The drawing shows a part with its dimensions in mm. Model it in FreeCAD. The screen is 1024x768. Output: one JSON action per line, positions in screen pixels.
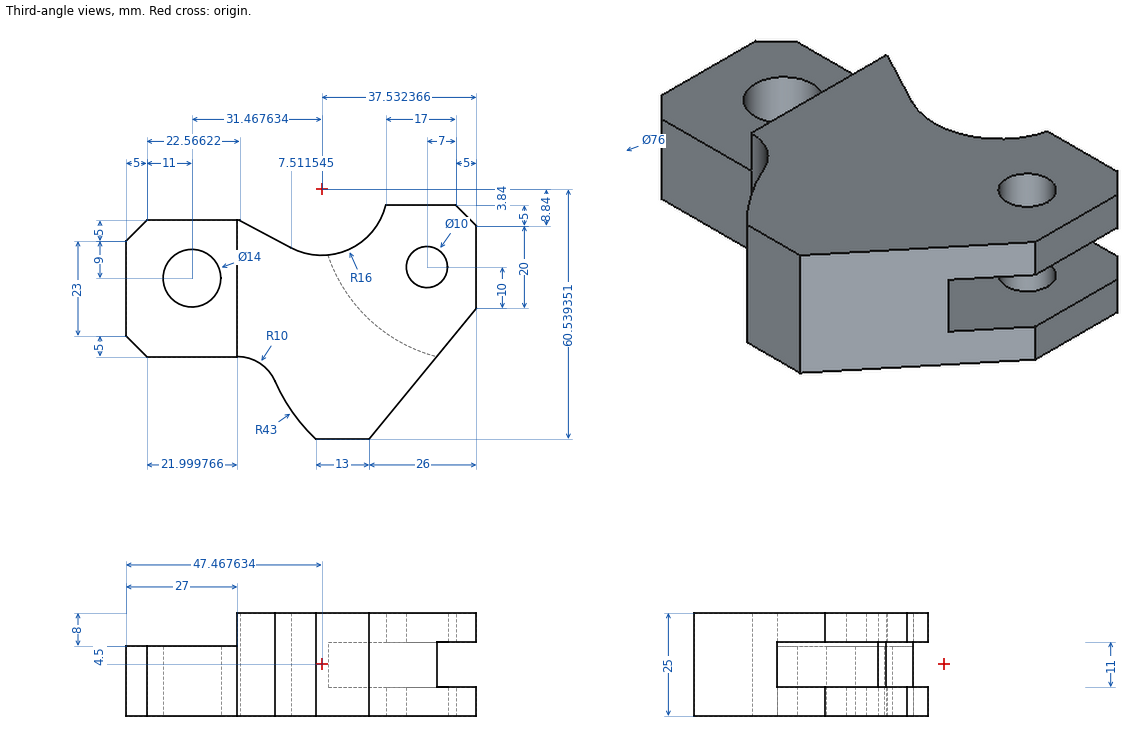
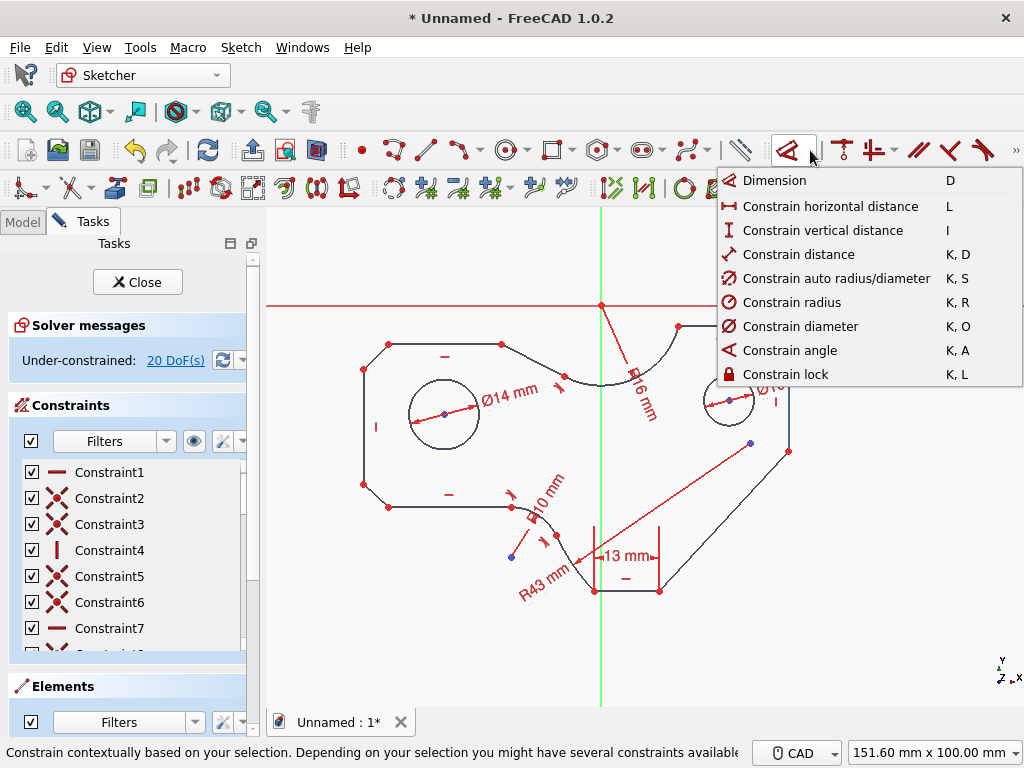
{"action": "left_click", "coordinate": [870, 230]}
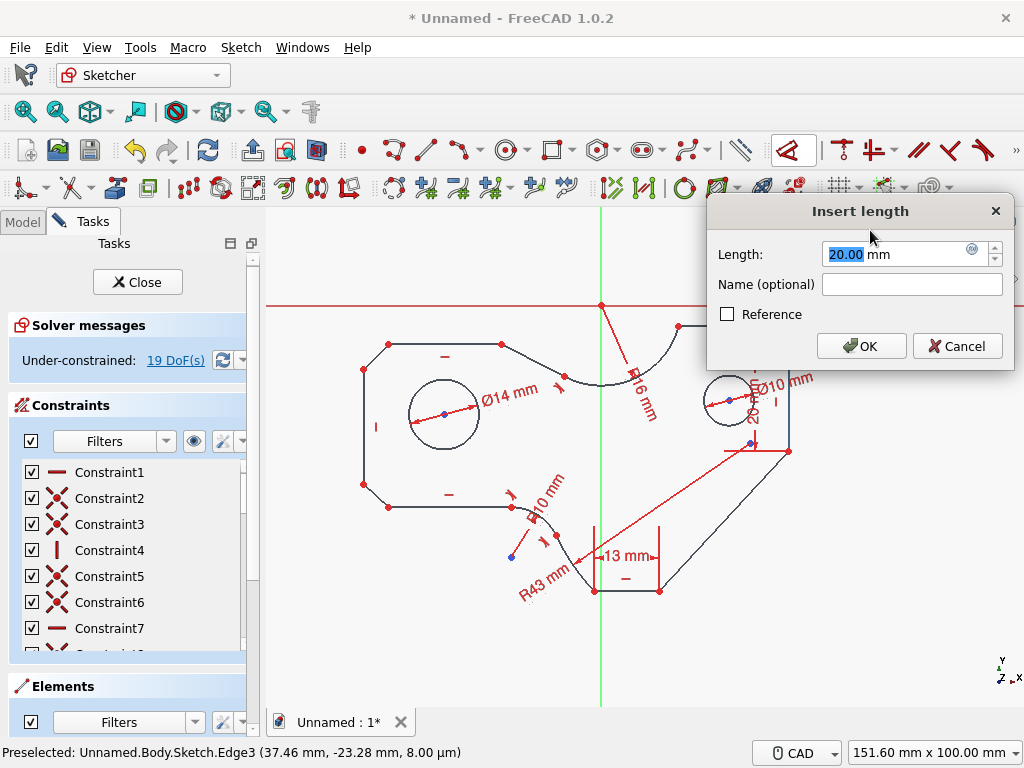
{"action": "type", "text": "20"}
{"action": "key", "text": "Return"}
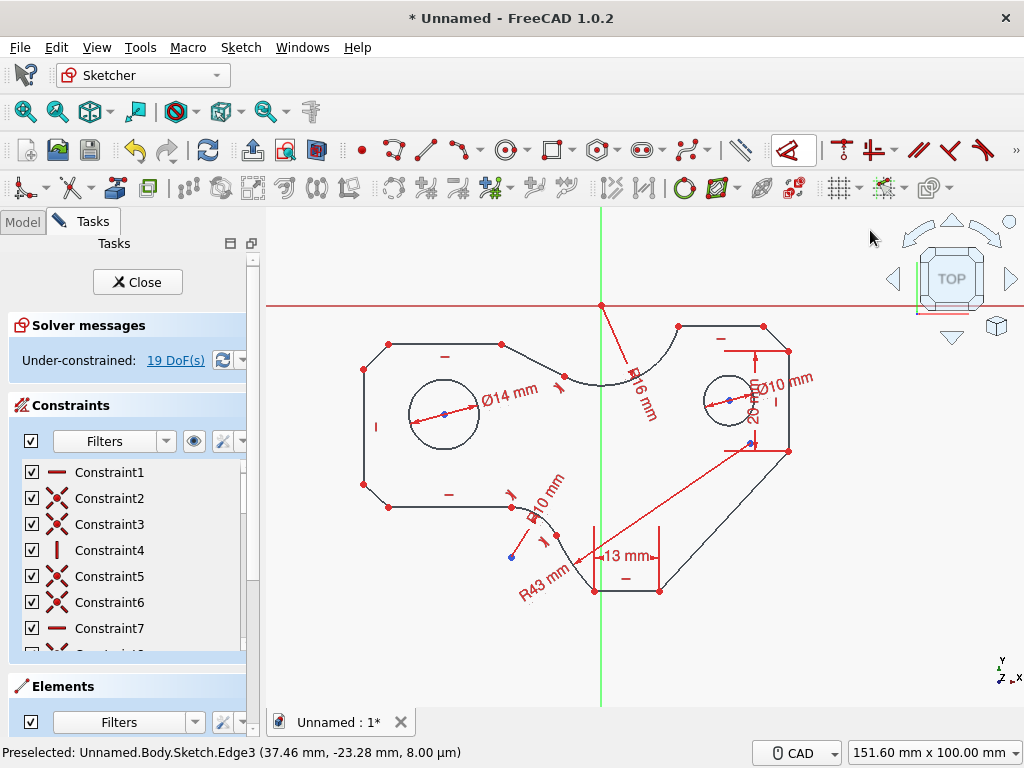
{"action": "left_click", "coordinate": [738, 326]}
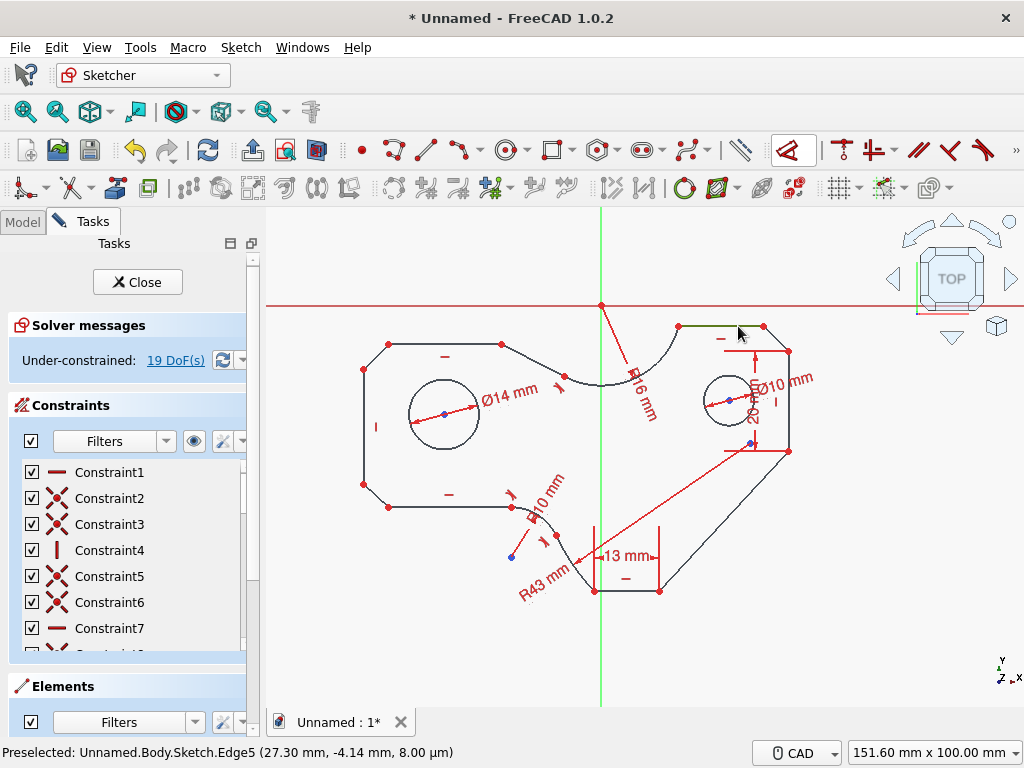
{"action": "left_click", "coordinate": [810, 150]}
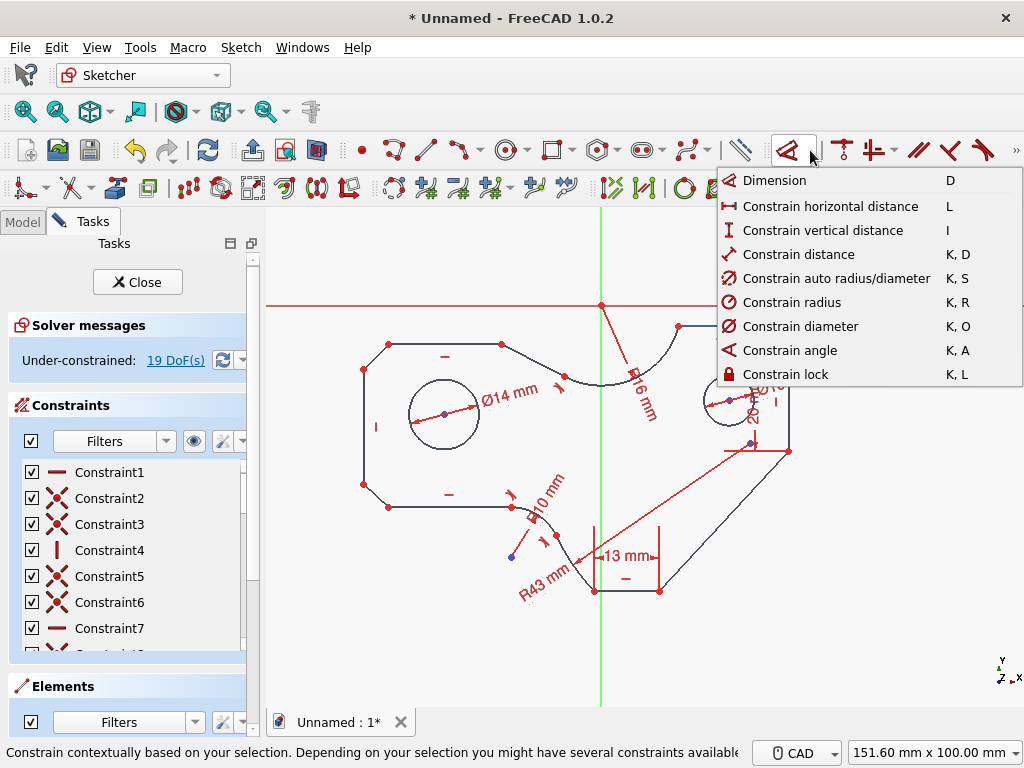
{"action": "left_click", "coordinate": [870, 206]}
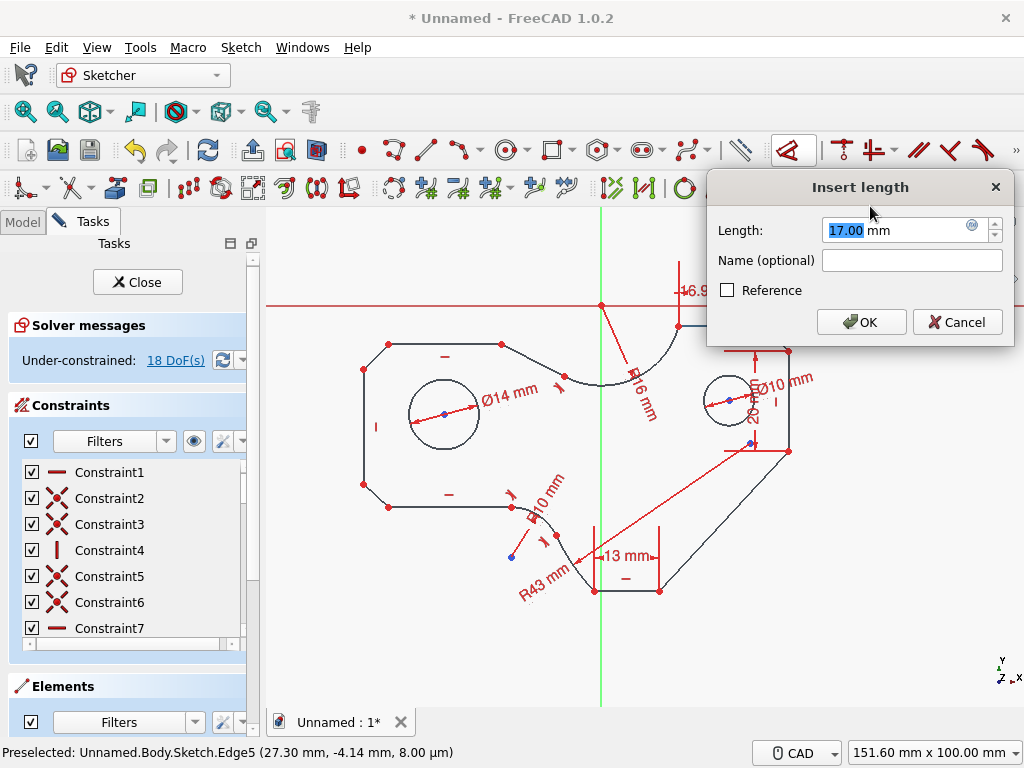
{"action": "type", "text": "17"}
{"action": "key", "text": "Return"}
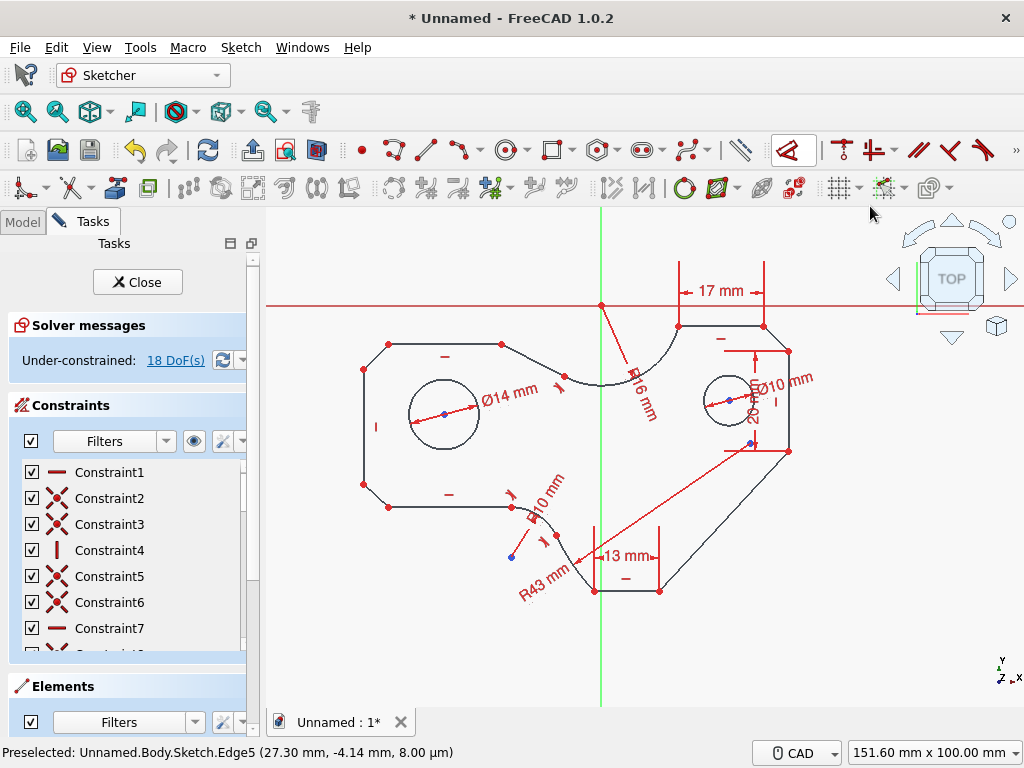
{"action": "left_click", "coordinate": [364, 404]}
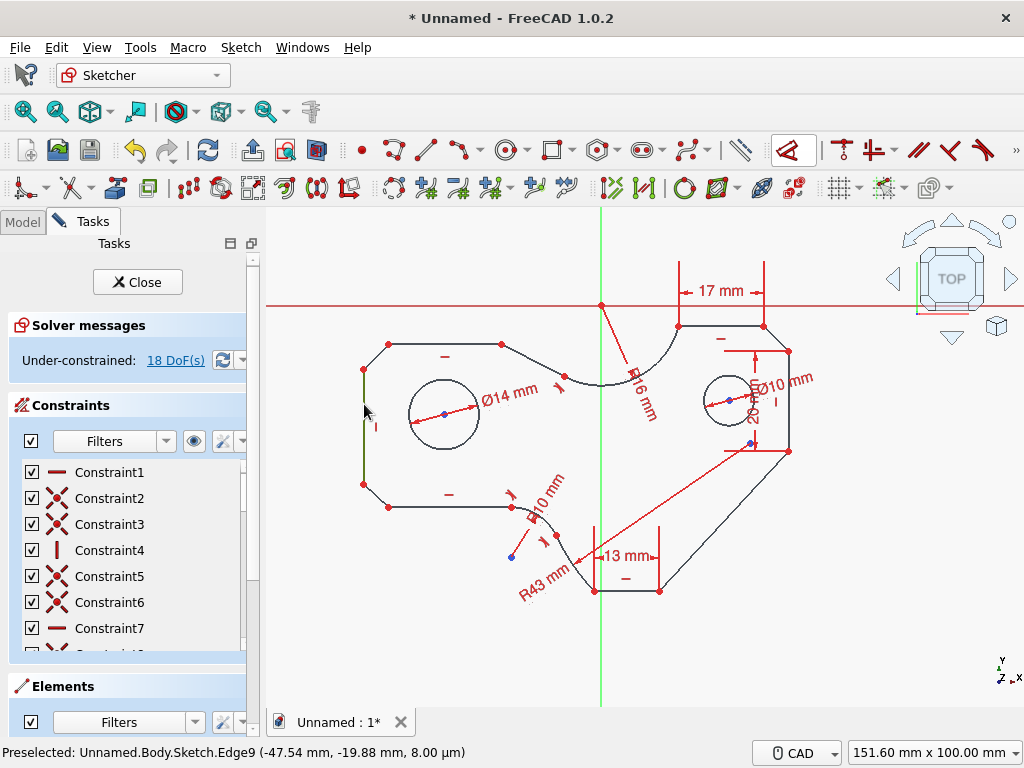
{"action": "key", "text": "i"}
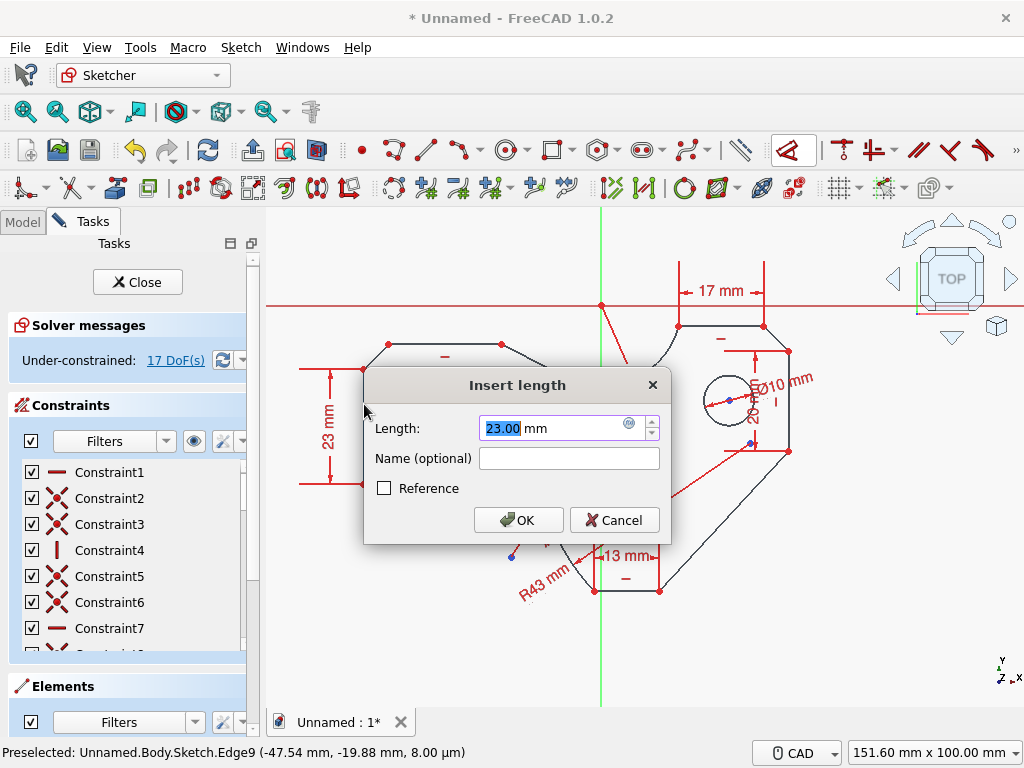
{"action": "type", "text": "23"}
{"action": "key", "text": "Return"}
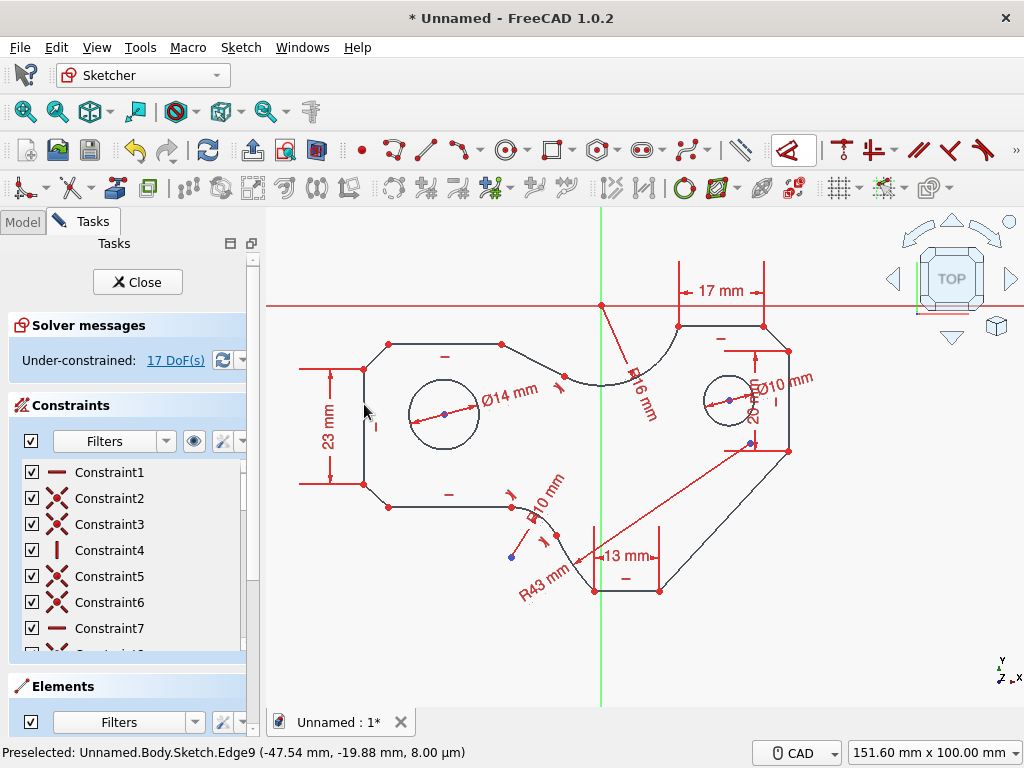
{"action": "scroll", "coordinate": [781, 344], "scroll_direction": "up", "scroll_amount": 3}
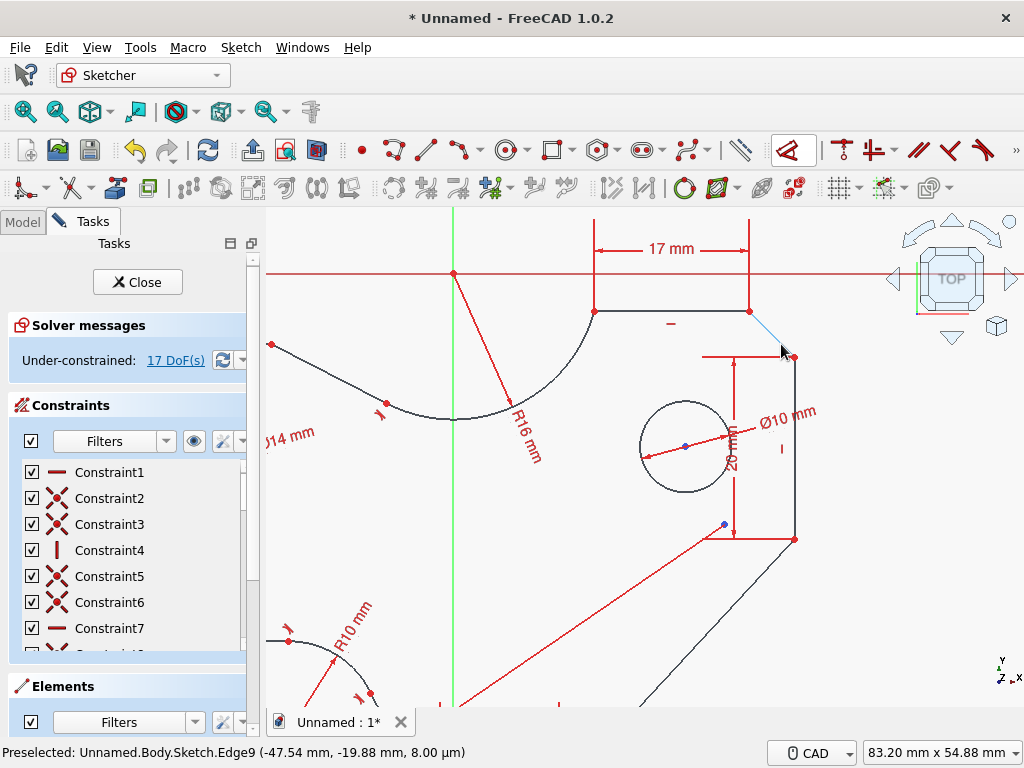
{"action": "left_click", "coordinate": [781, 343]}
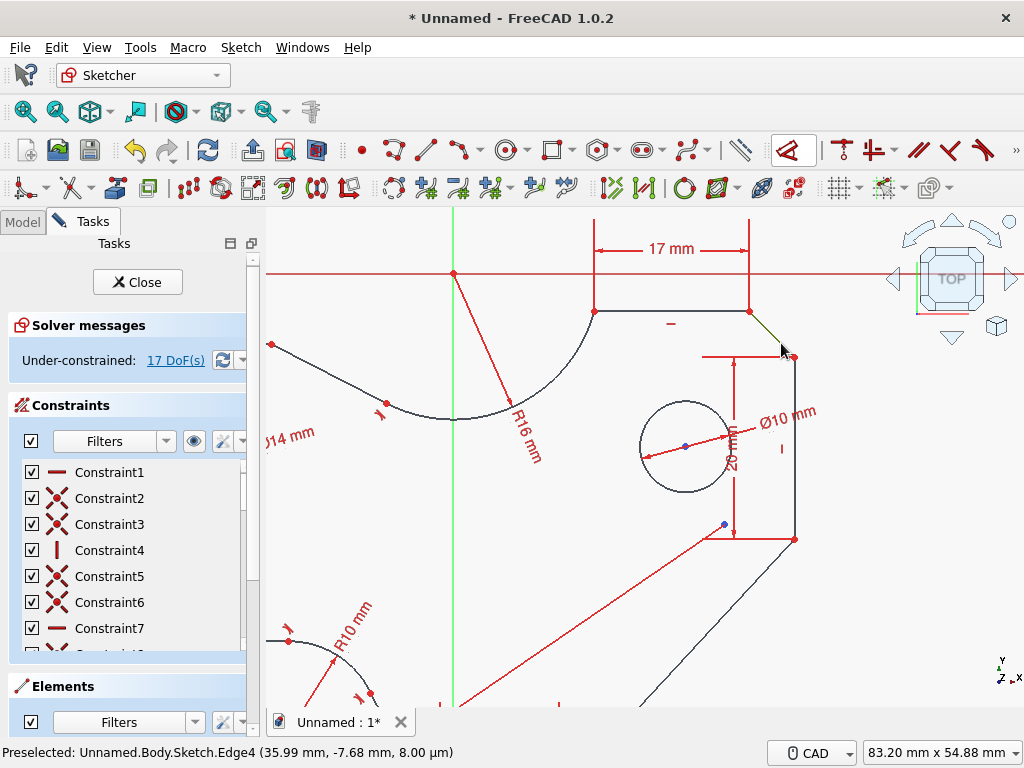
{"action": "left_click", "coordinate": [810, 150]}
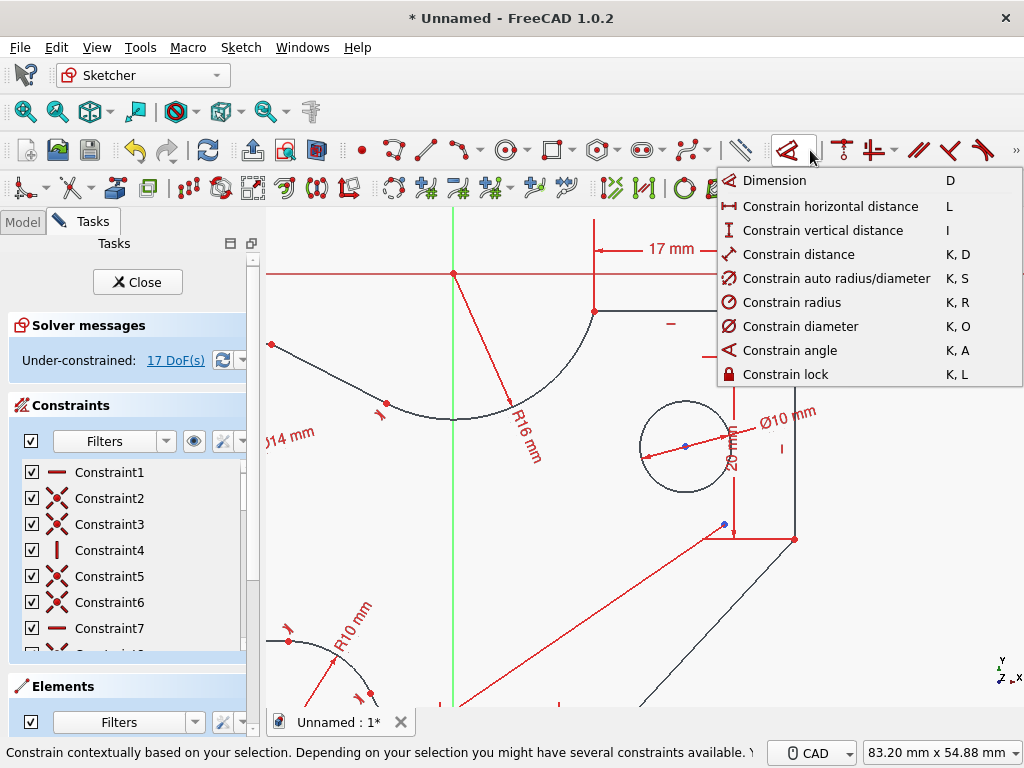
{"action": "left_click", "coordinate": [870, 206]}